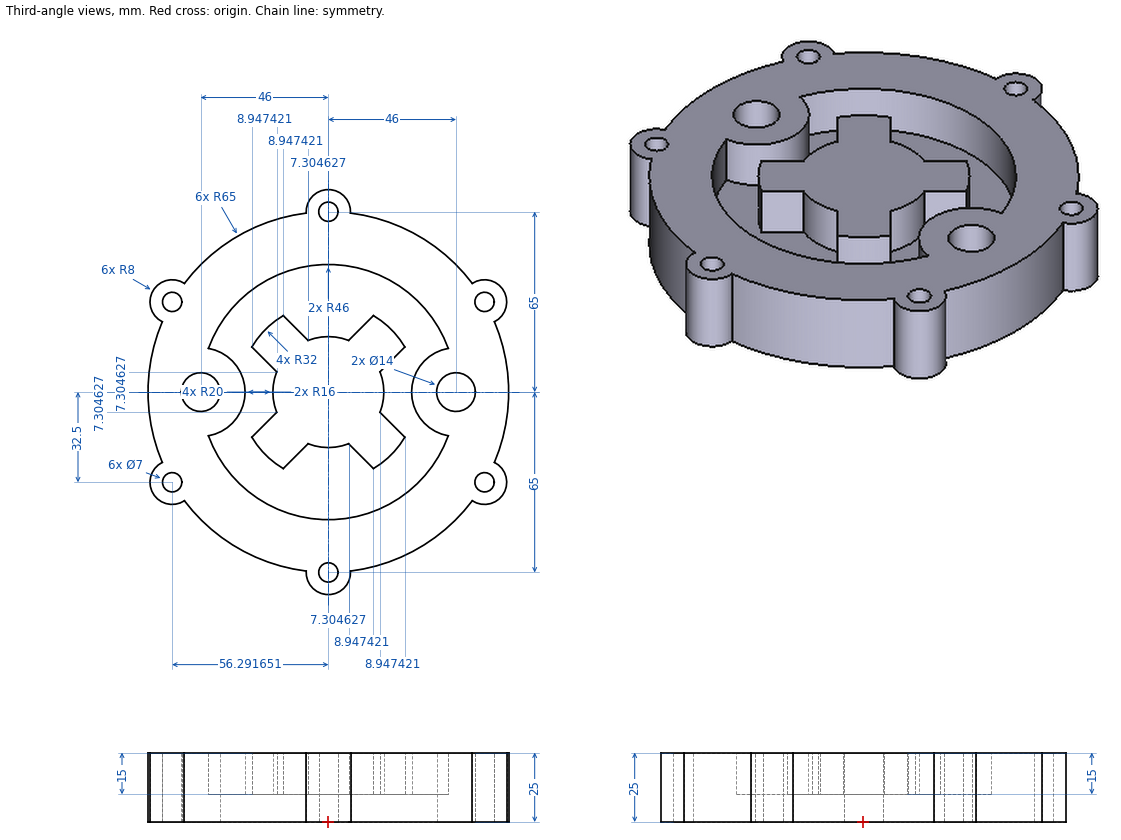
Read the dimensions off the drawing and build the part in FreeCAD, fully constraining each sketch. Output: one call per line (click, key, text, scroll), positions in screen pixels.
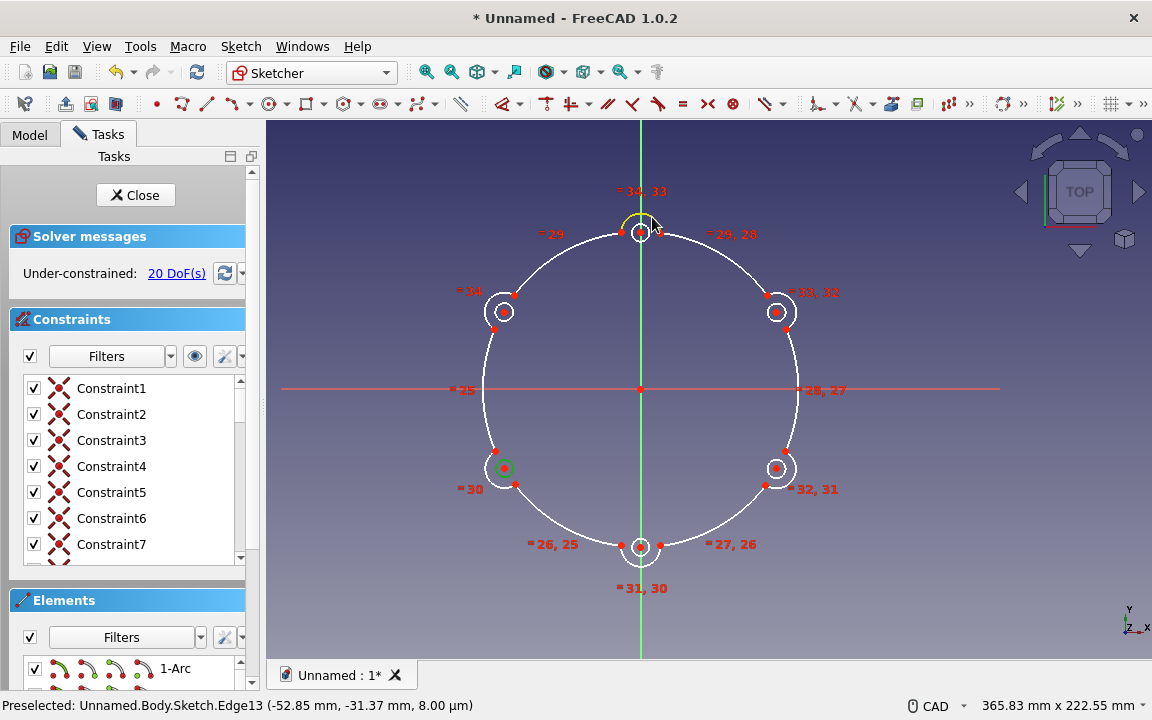
scroll(647, 553, up, 5)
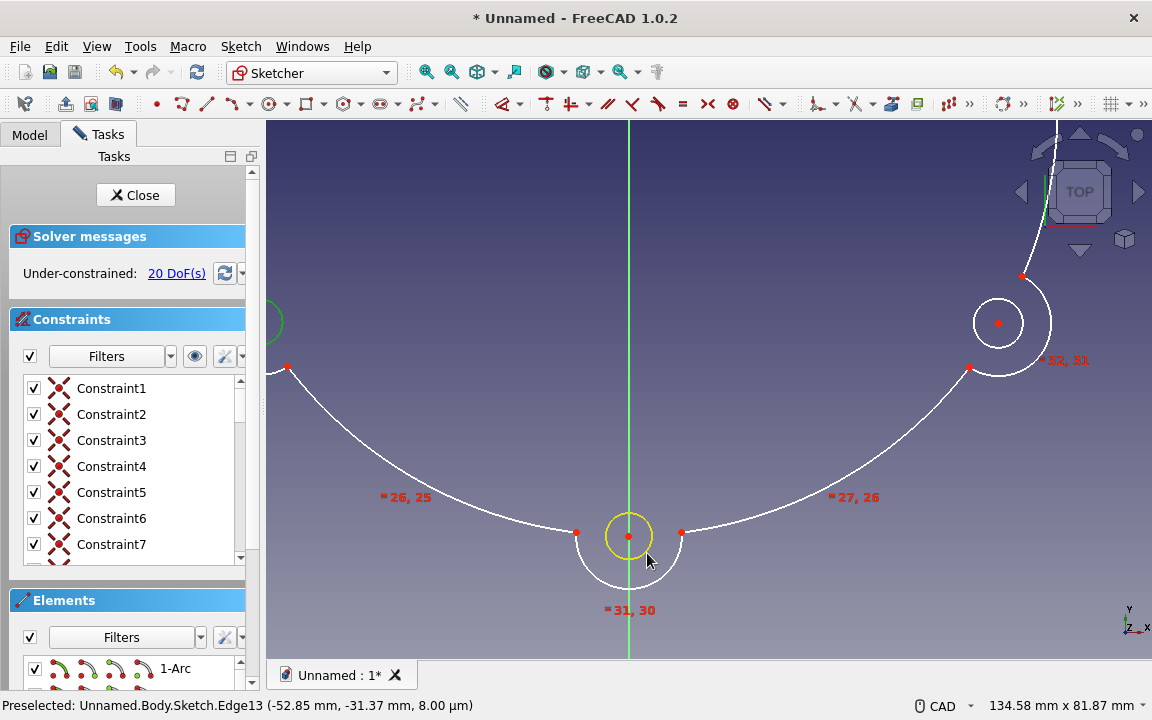
click(645, 552)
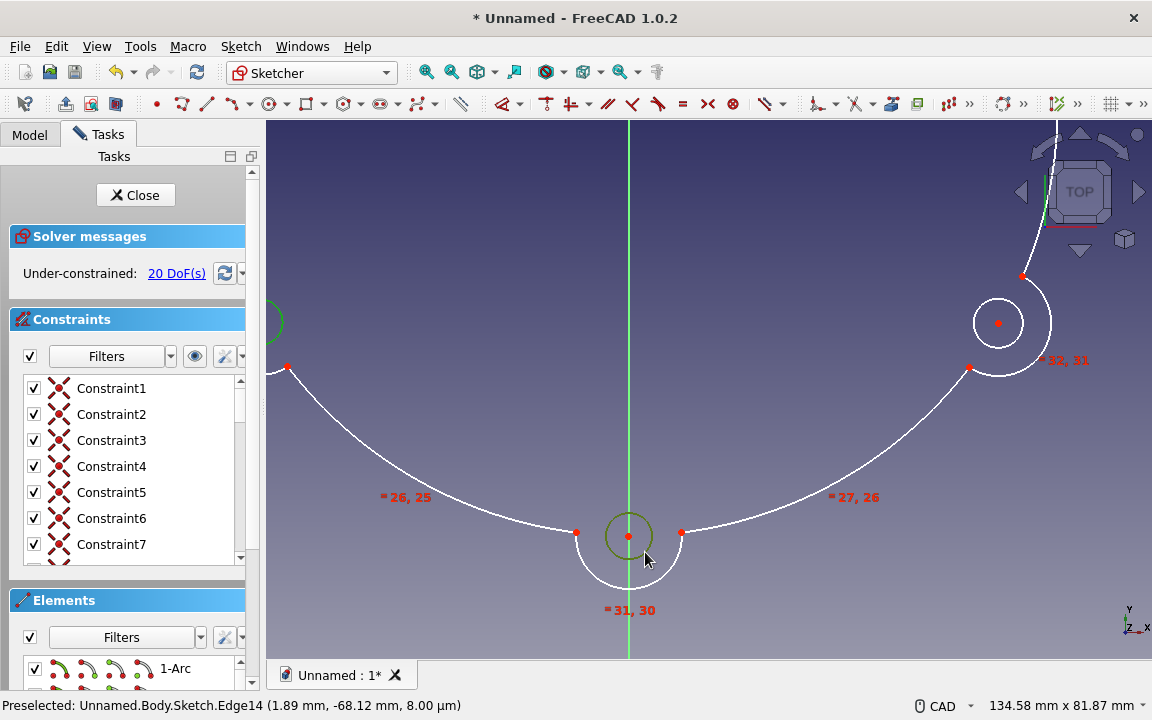
click(981, 306)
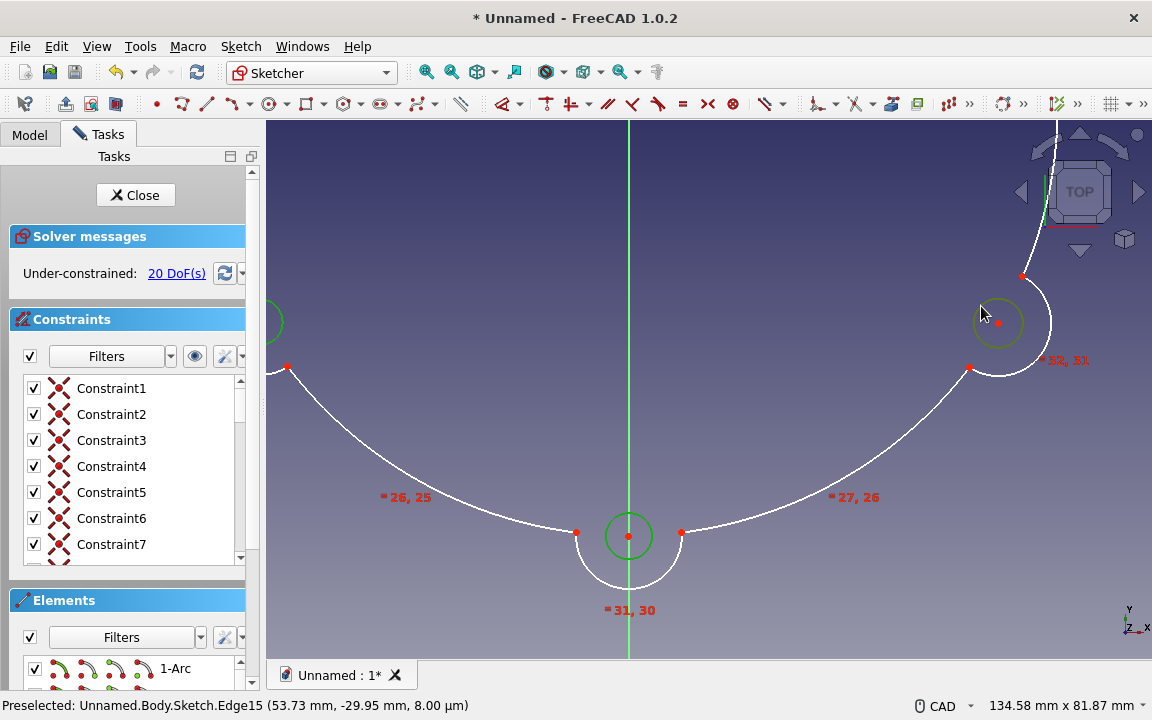
scroll(647, 554, down, 5)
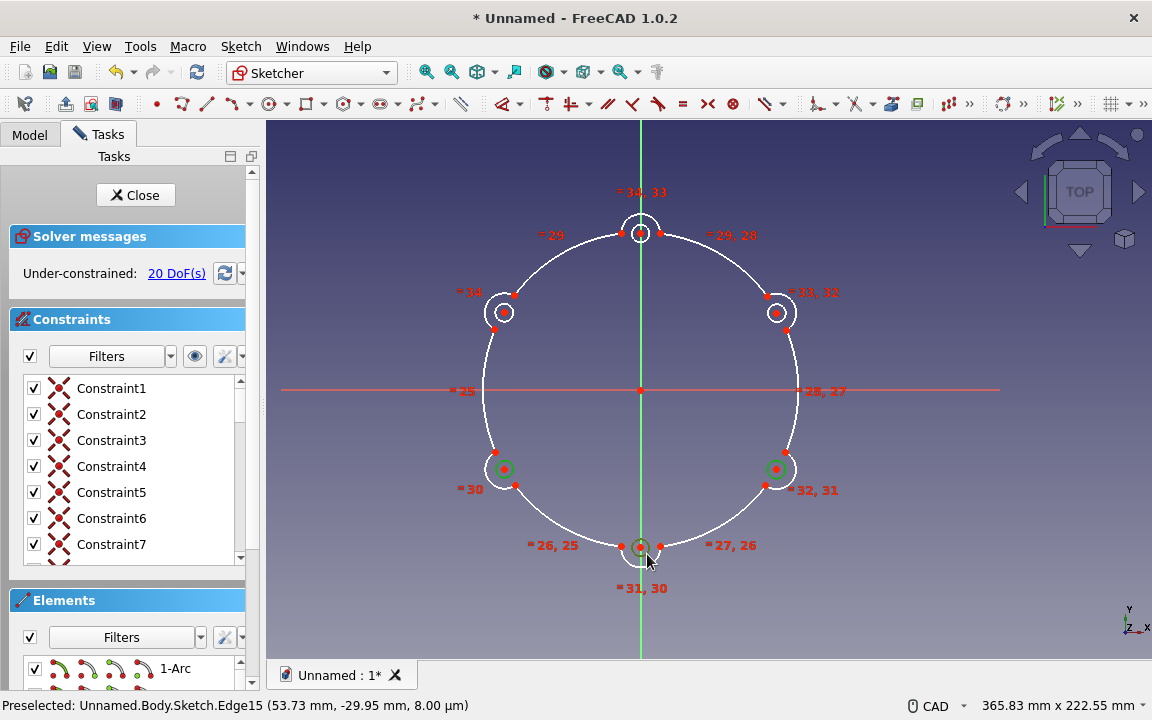
scroll(511, 306, up, 3)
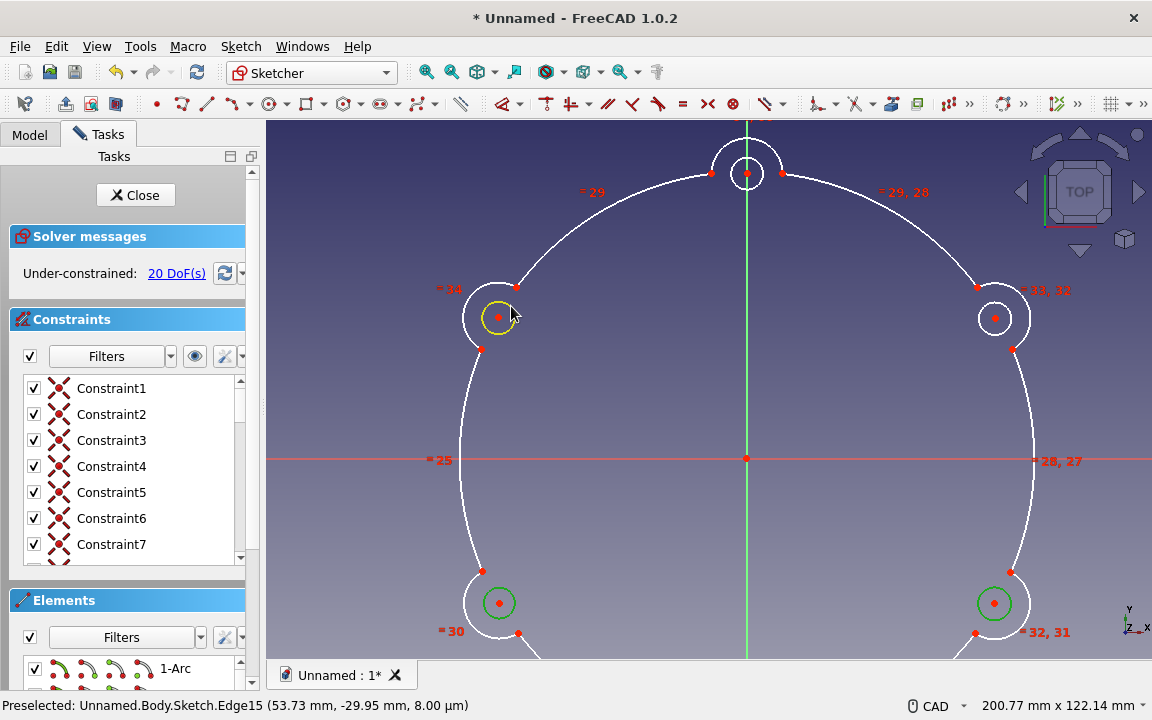
click(510, 306)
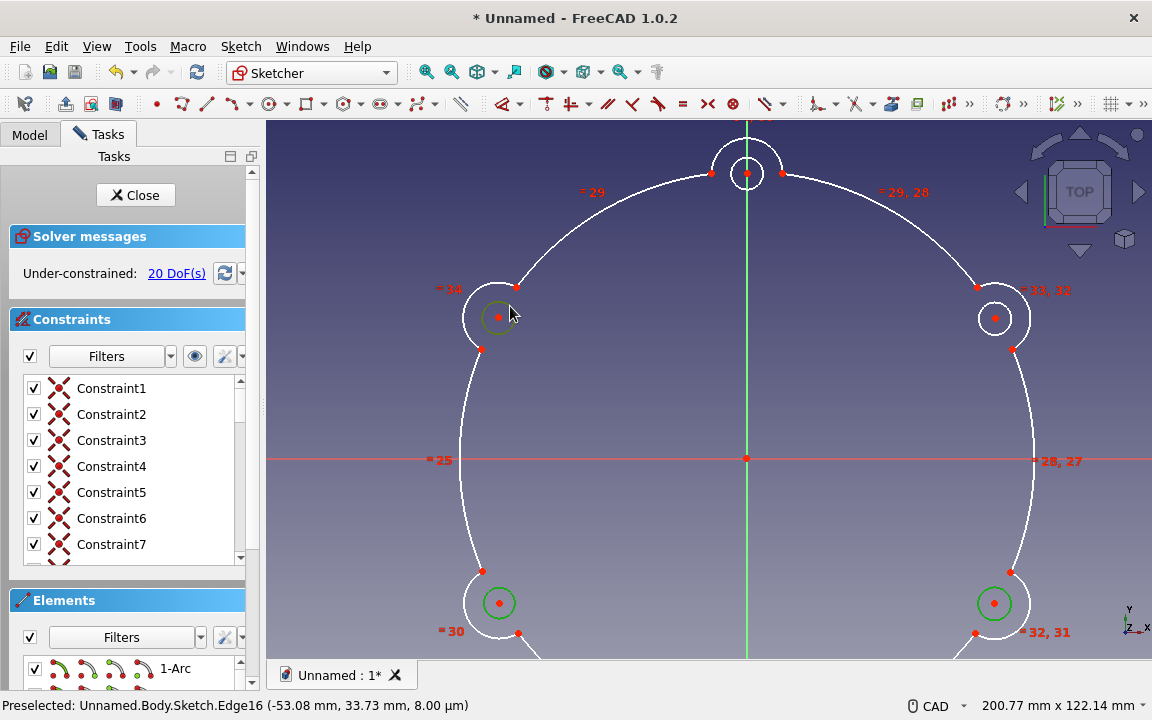
click(984, 307)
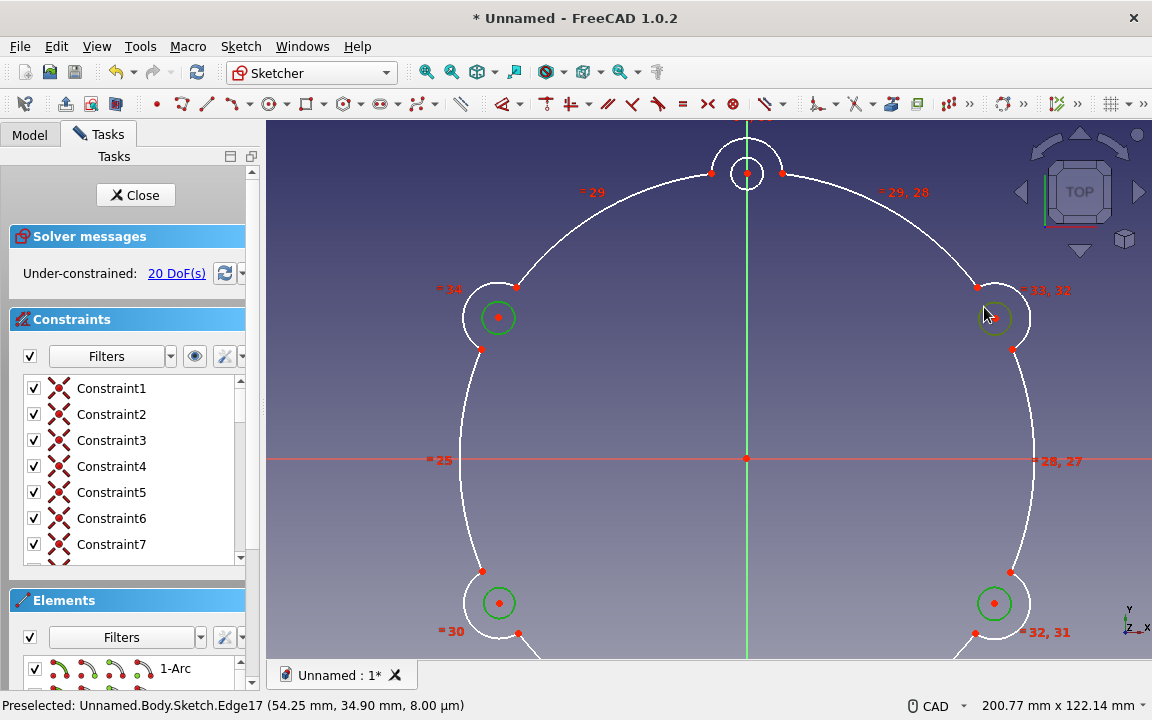
click(758, 162)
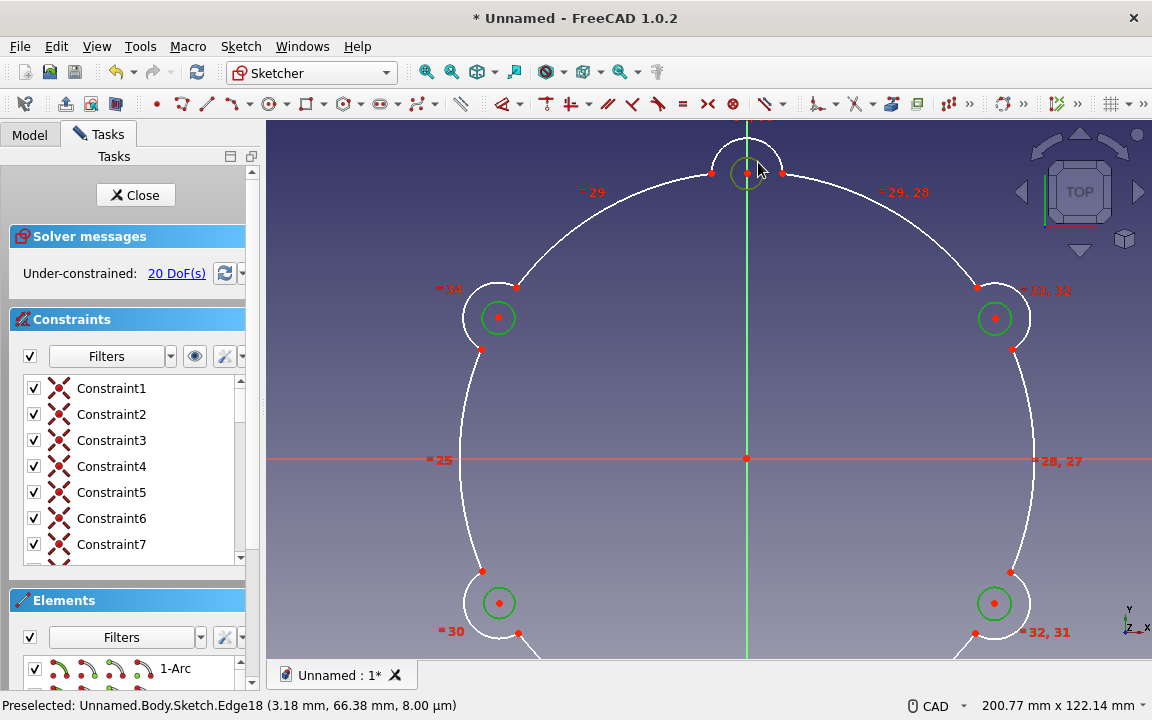
click(683, 104)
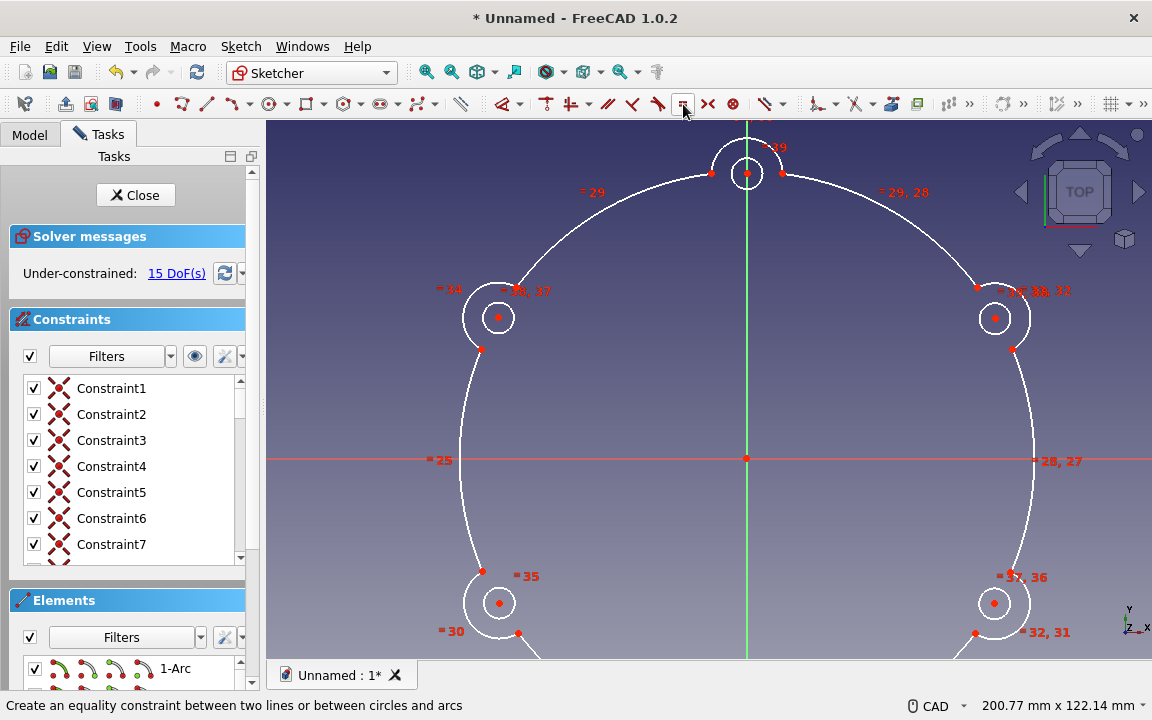
scroll(511, 305, down, 3)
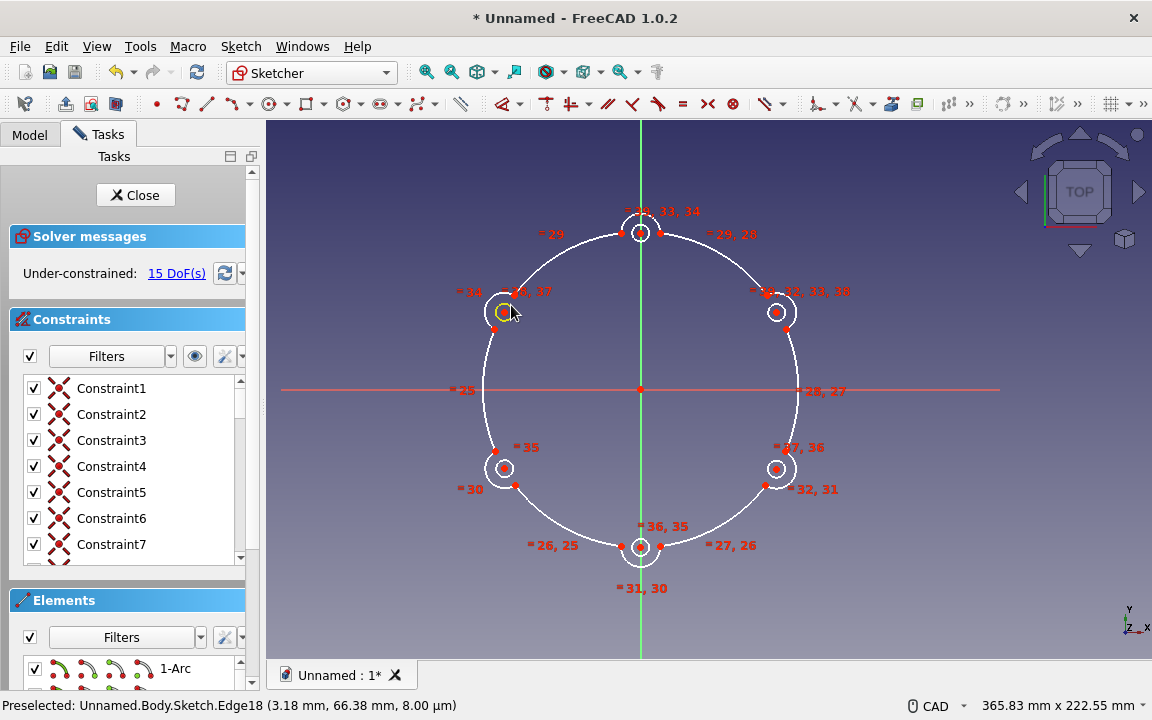
click(641, 547)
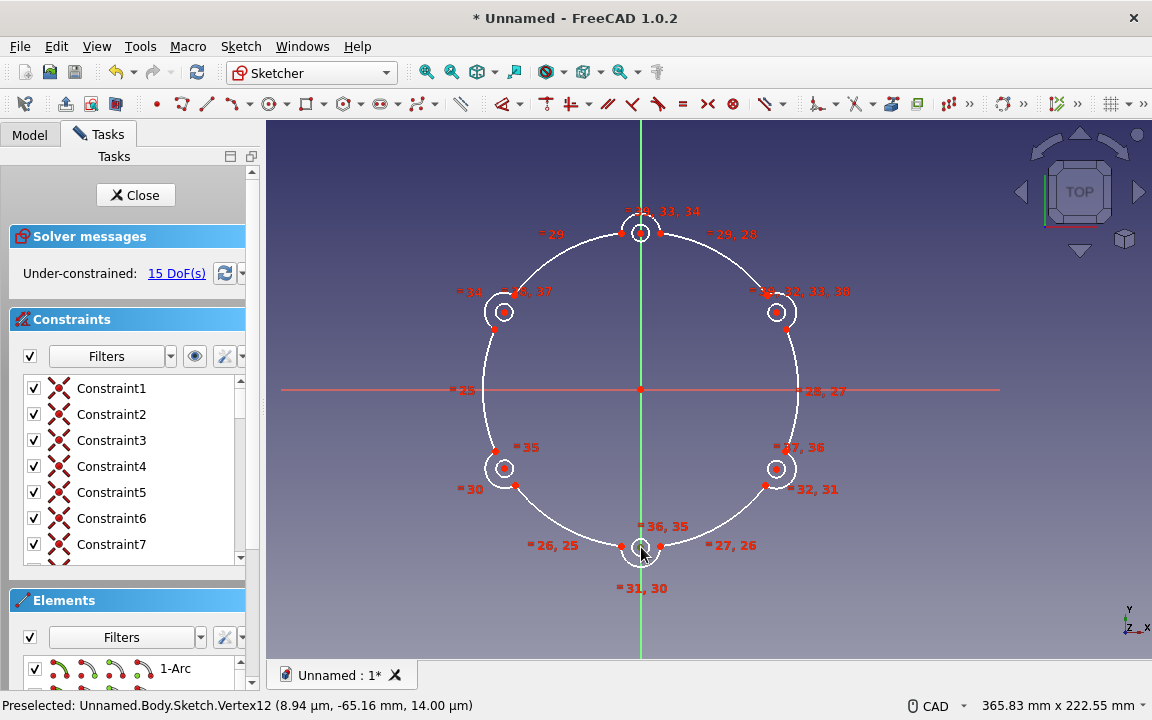
click(641, 493)